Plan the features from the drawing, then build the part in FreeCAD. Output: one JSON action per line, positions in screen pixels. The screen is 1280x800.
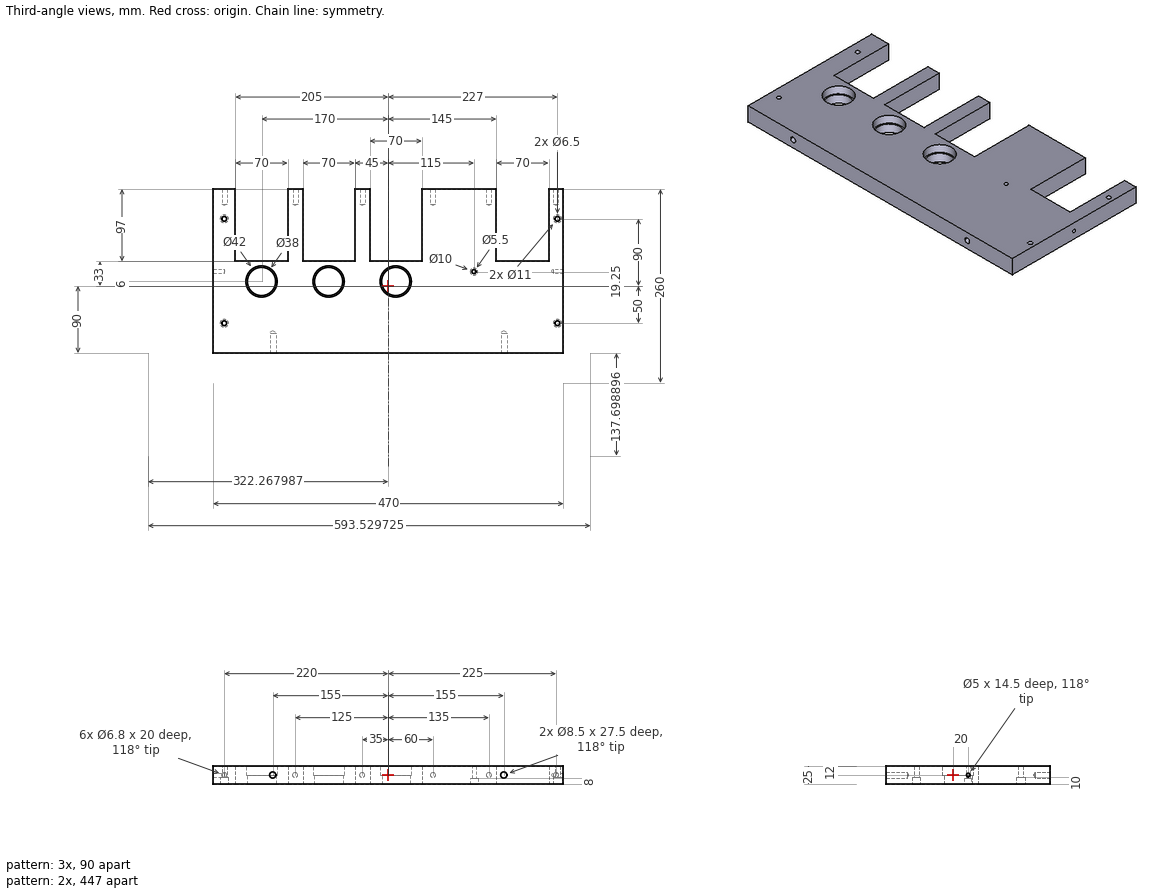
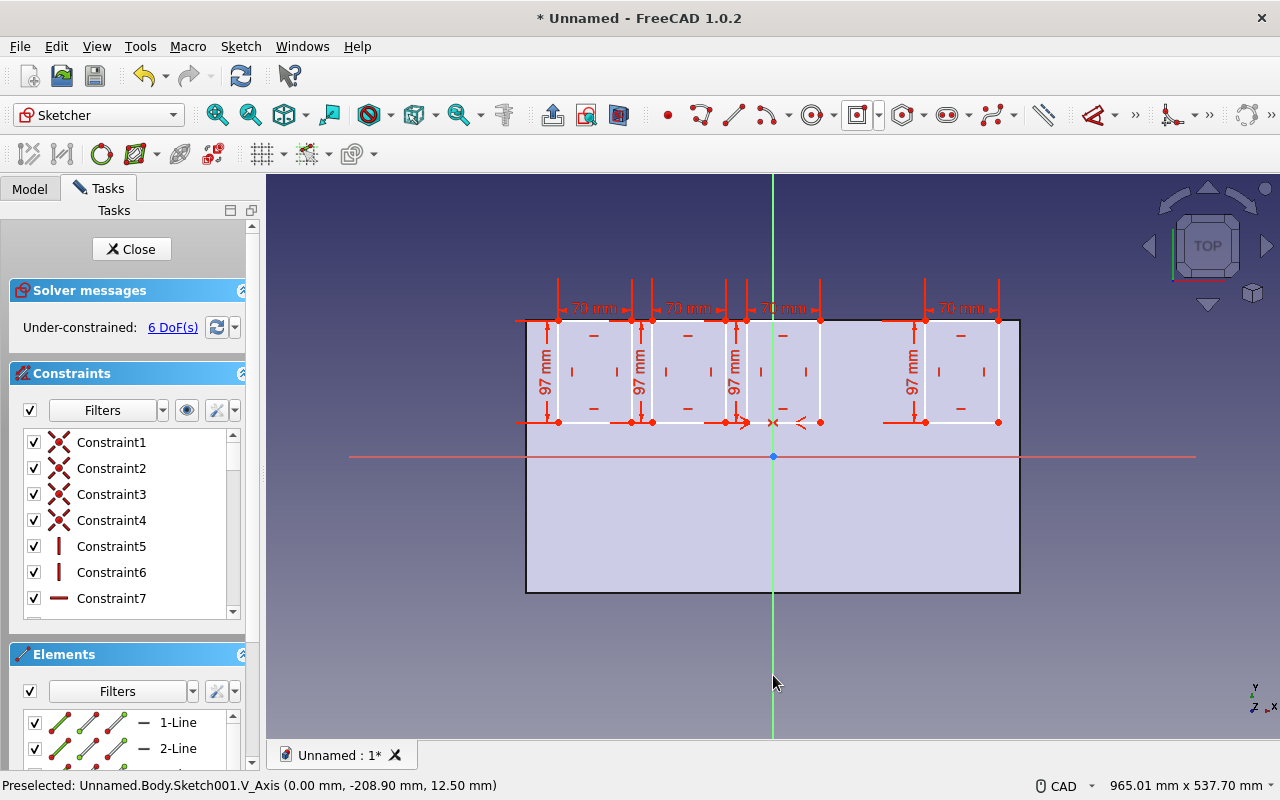
{"action": "left_click", "coordinate": [1092, 116]}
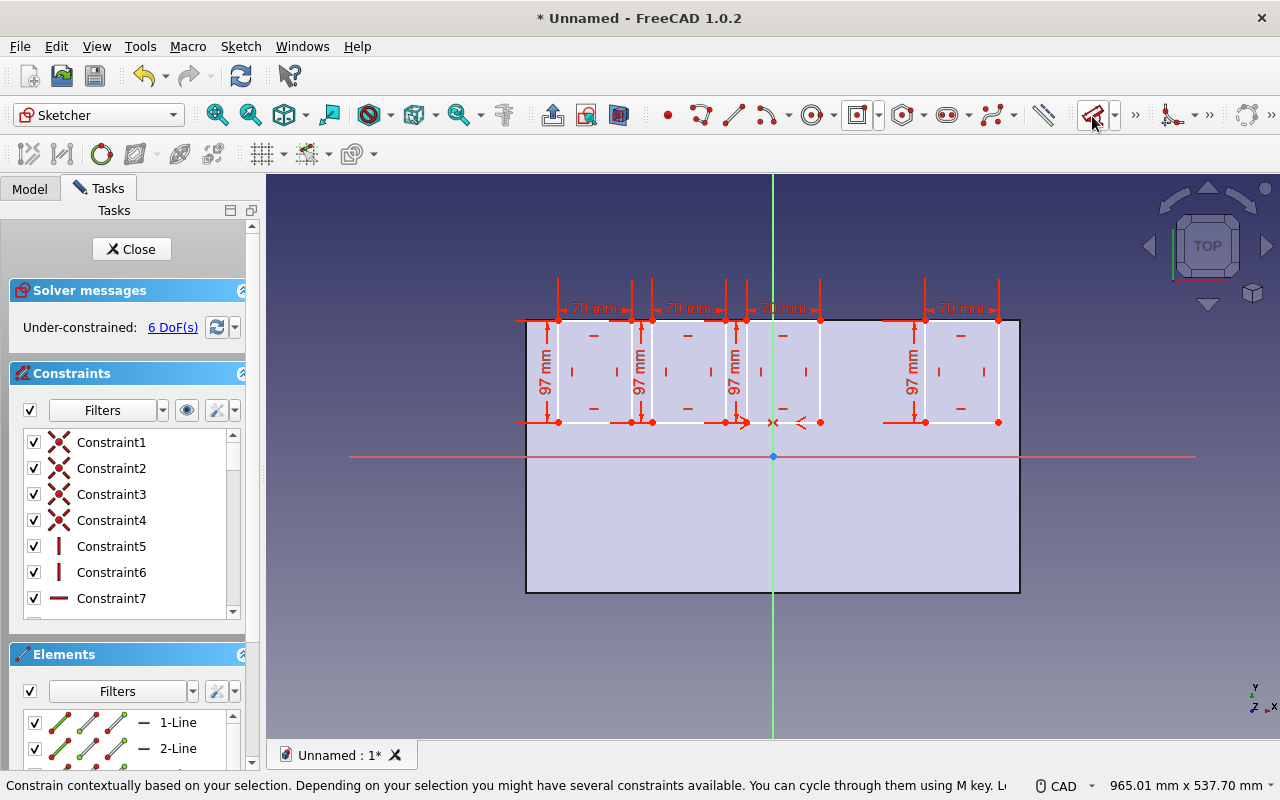
{"action": "left_click", "coordinate": [558, 423]}
{"action": "left_click", "coordinate": [524, 440]}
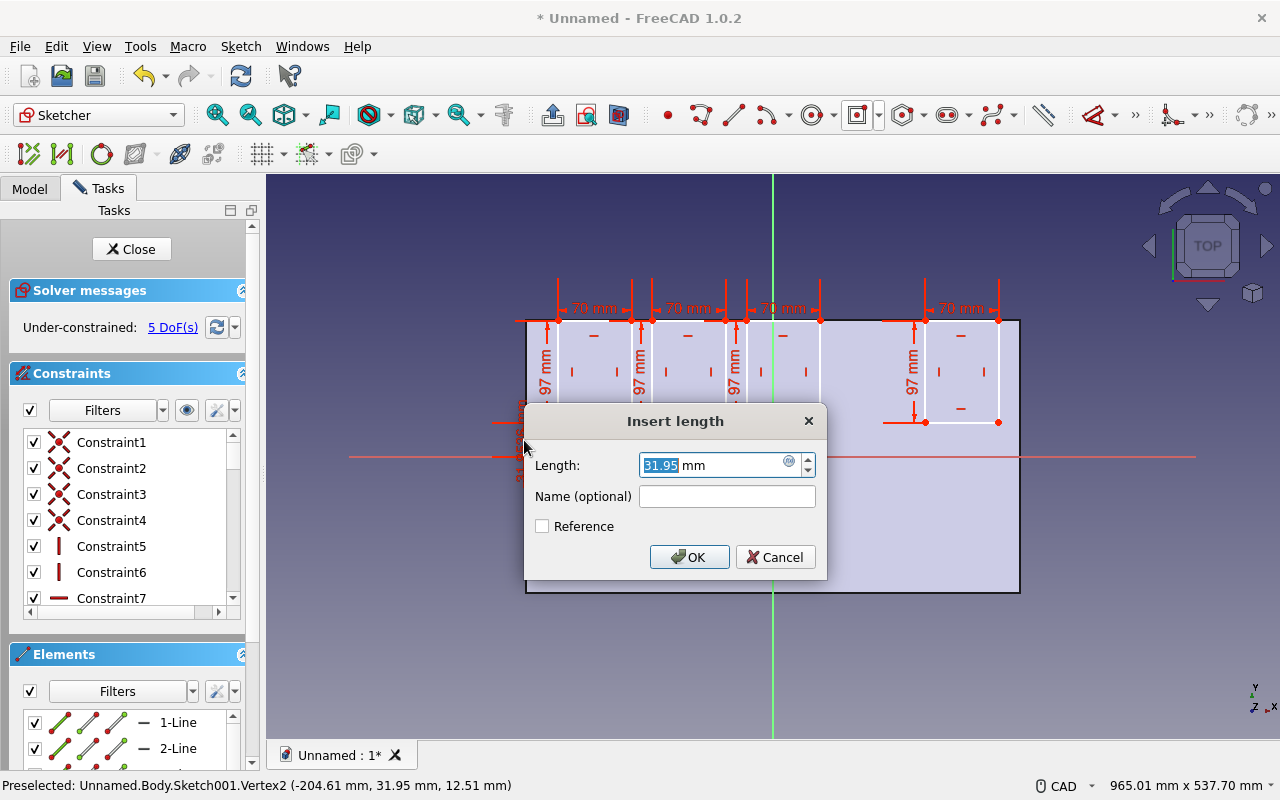
{"action": "type", "text": "33"}
{"action": "key", "text": "Return"}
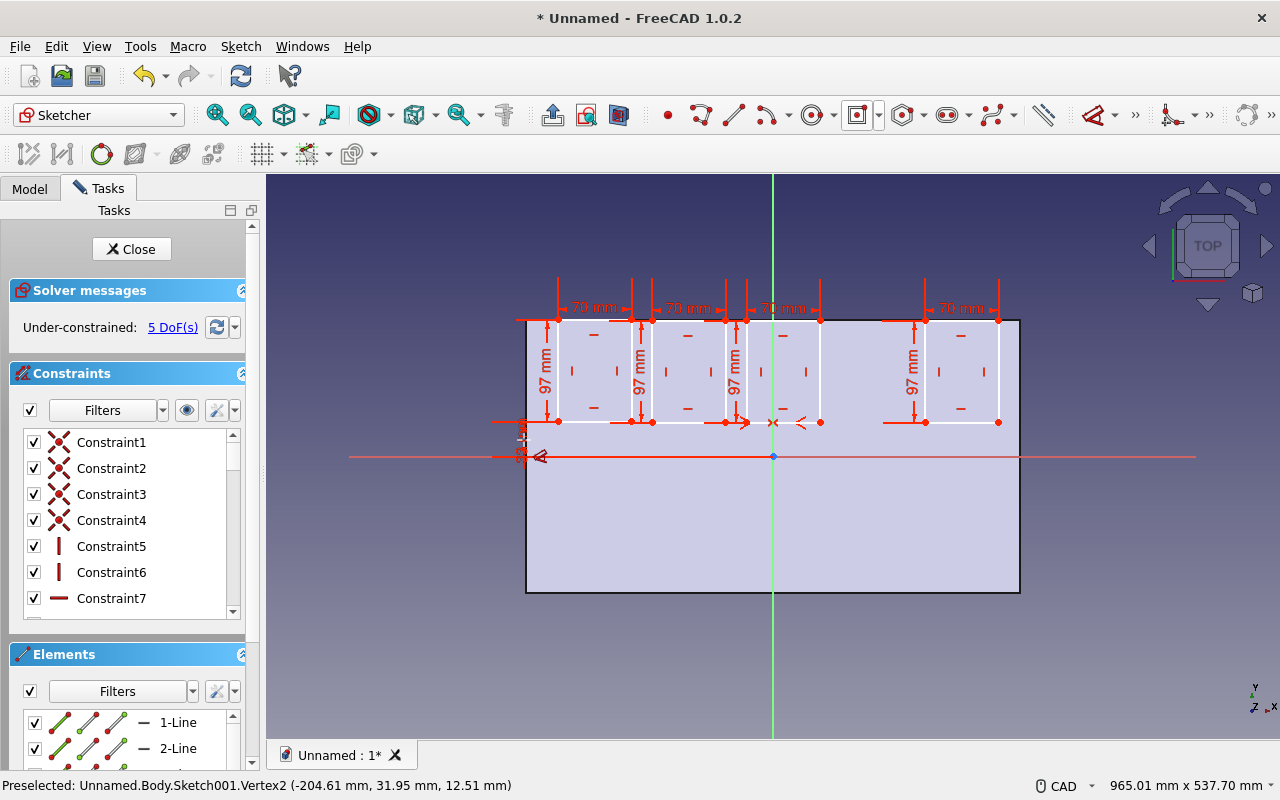
{"action": "left_click", "coordinate": [652, 423]}
{"action": "left_click", "coordinate": [618, 440]}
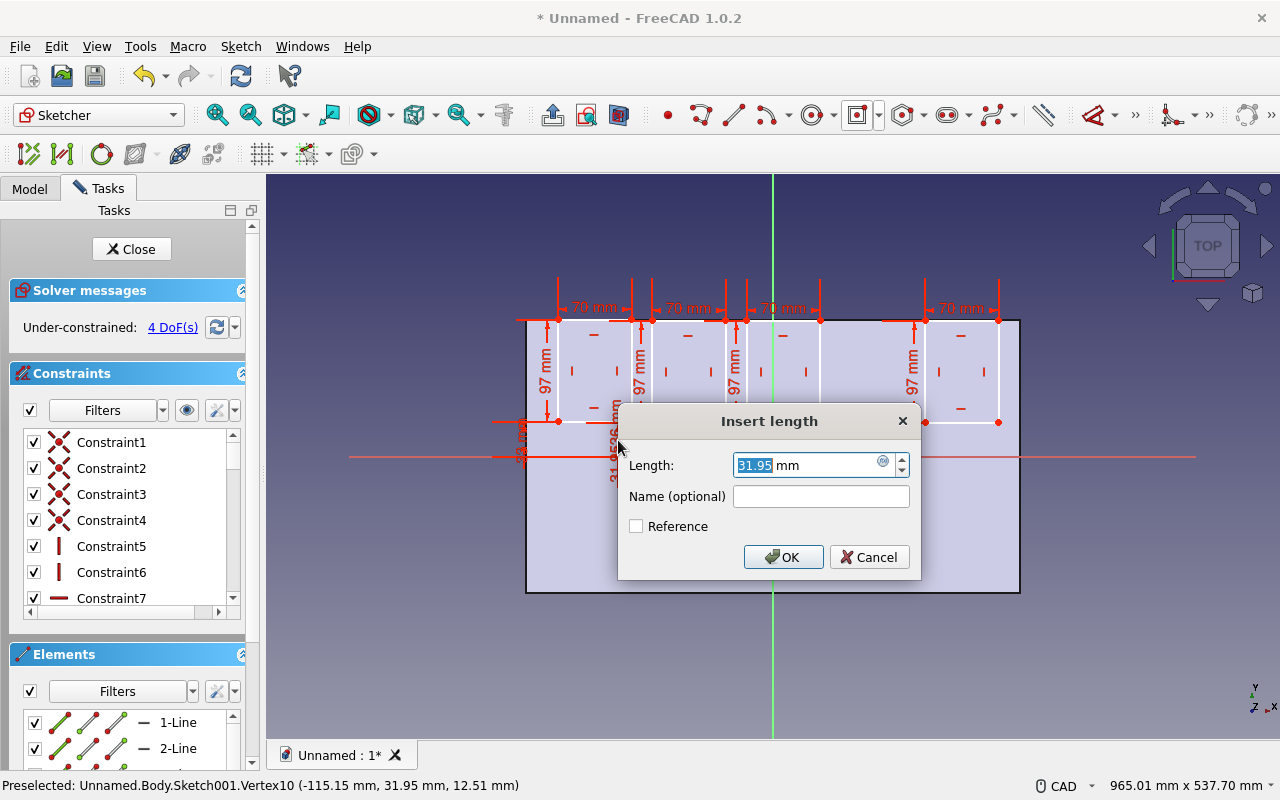
{"action": "type", "text": "33"}
{"action": "key", "text": "Return"}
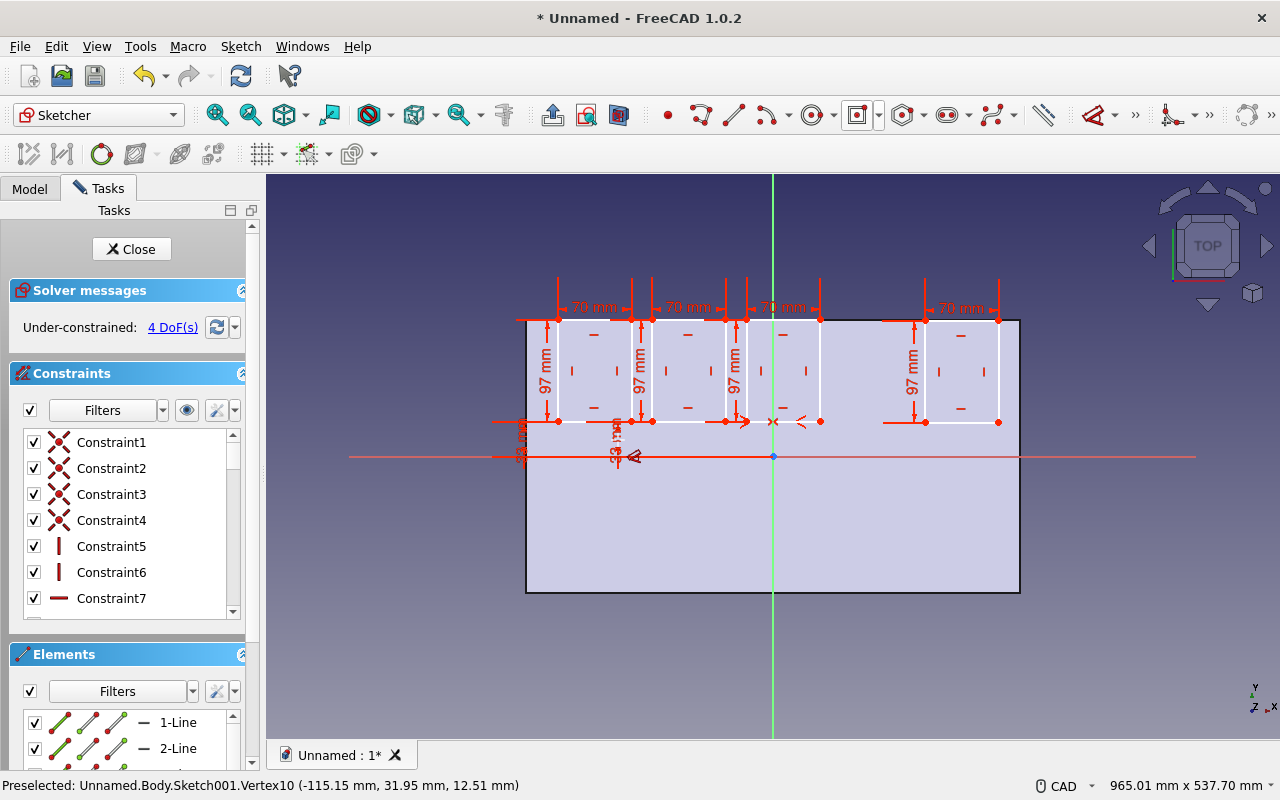
{"action": "left_click", "coordinate": [726, 422]}
{"action": "left_click", "coordinate": [749, 490]}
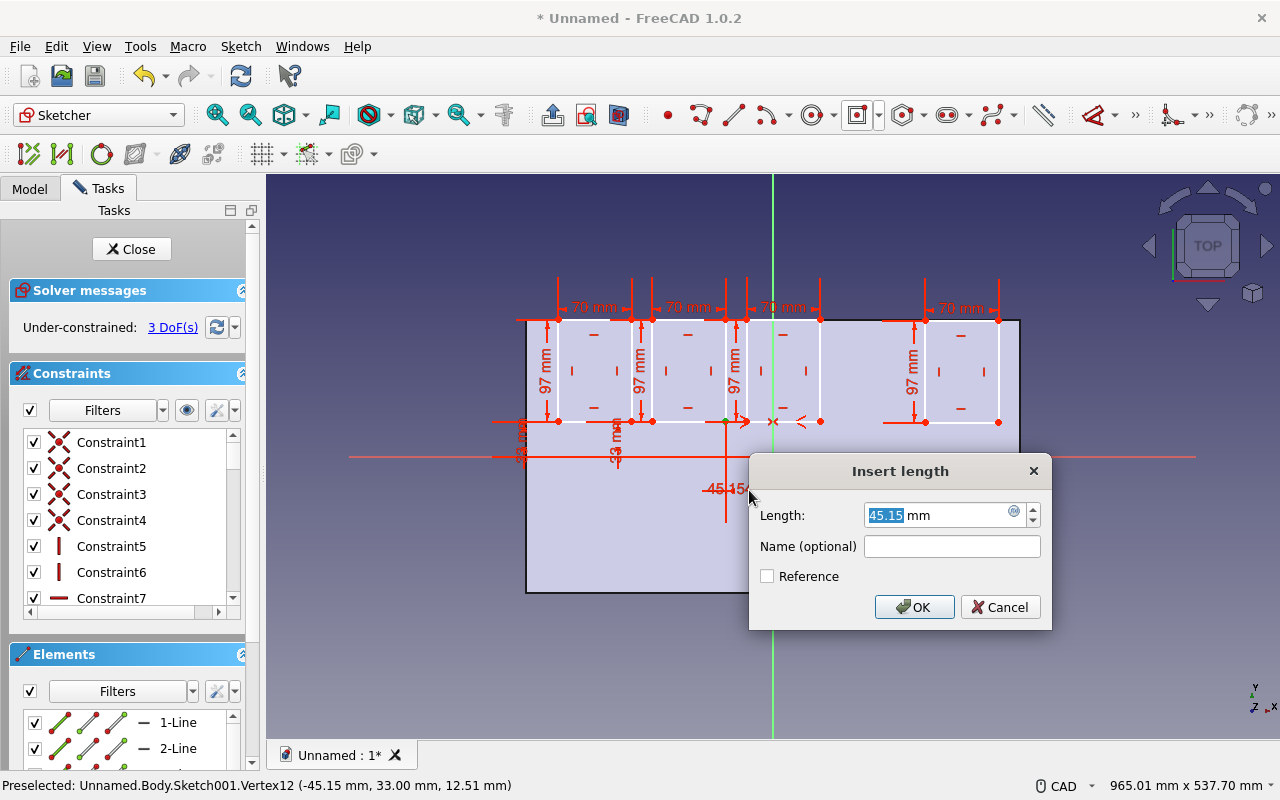
{"action": "type", "text": "45"}
{"action": "key", "text": "Return"}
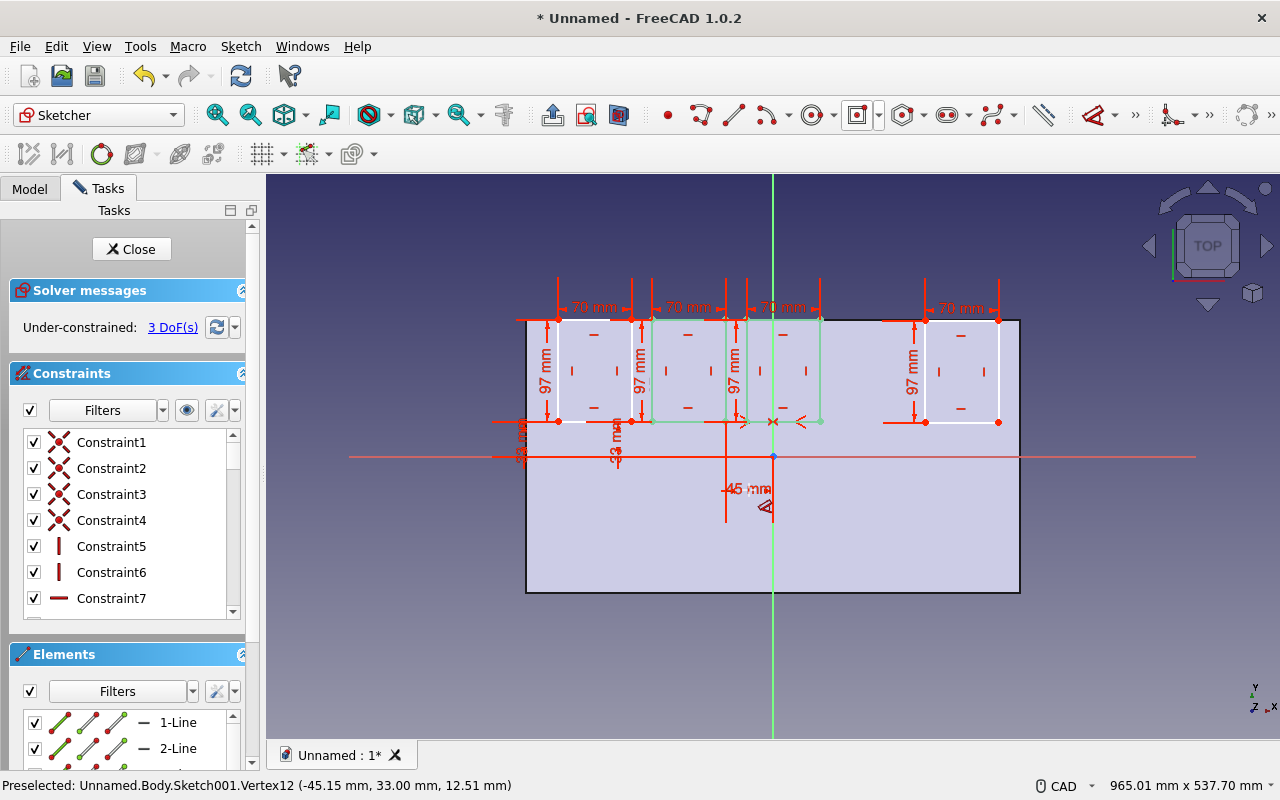
{"action": "left_click", "coordinate": [925, 423]}
{"action": "left_click", "coordinate": [959, 440]}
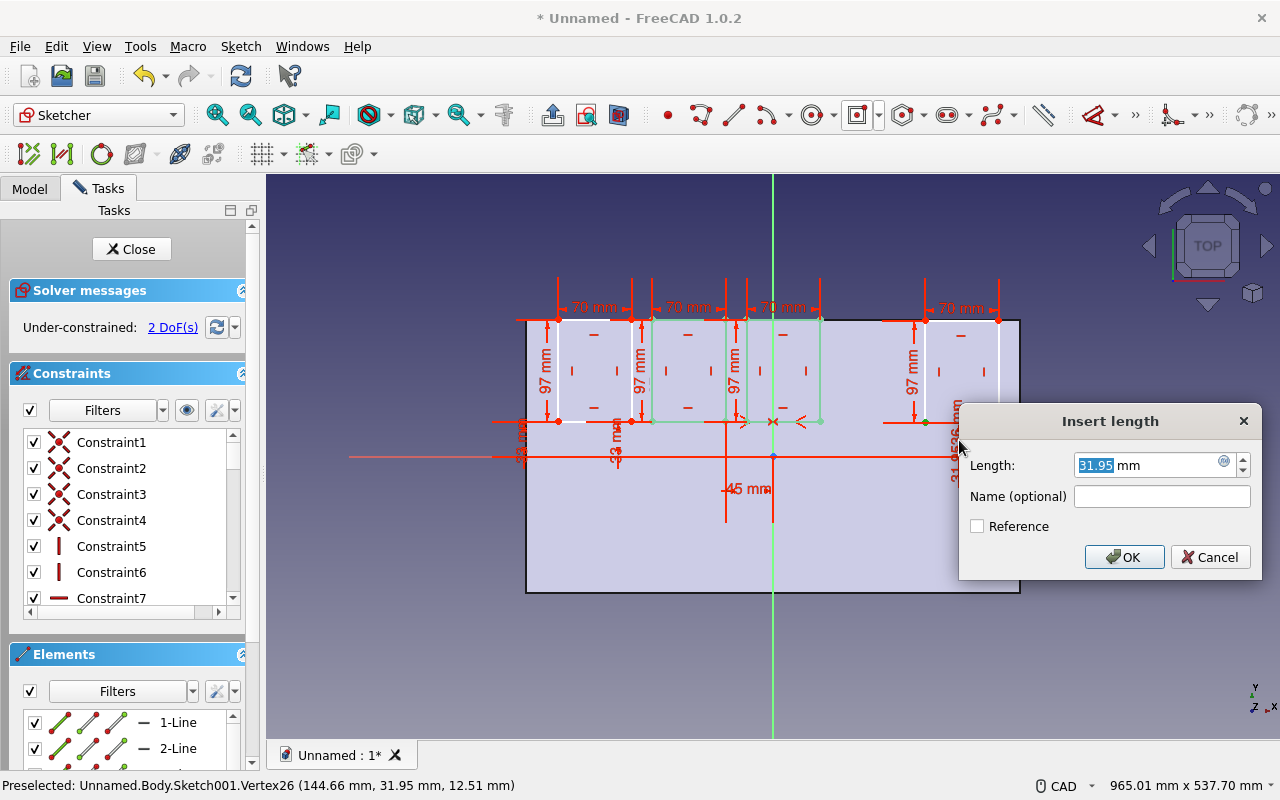
{"action": "type", "text": "33"}
{"action": "key", "text": "Return"}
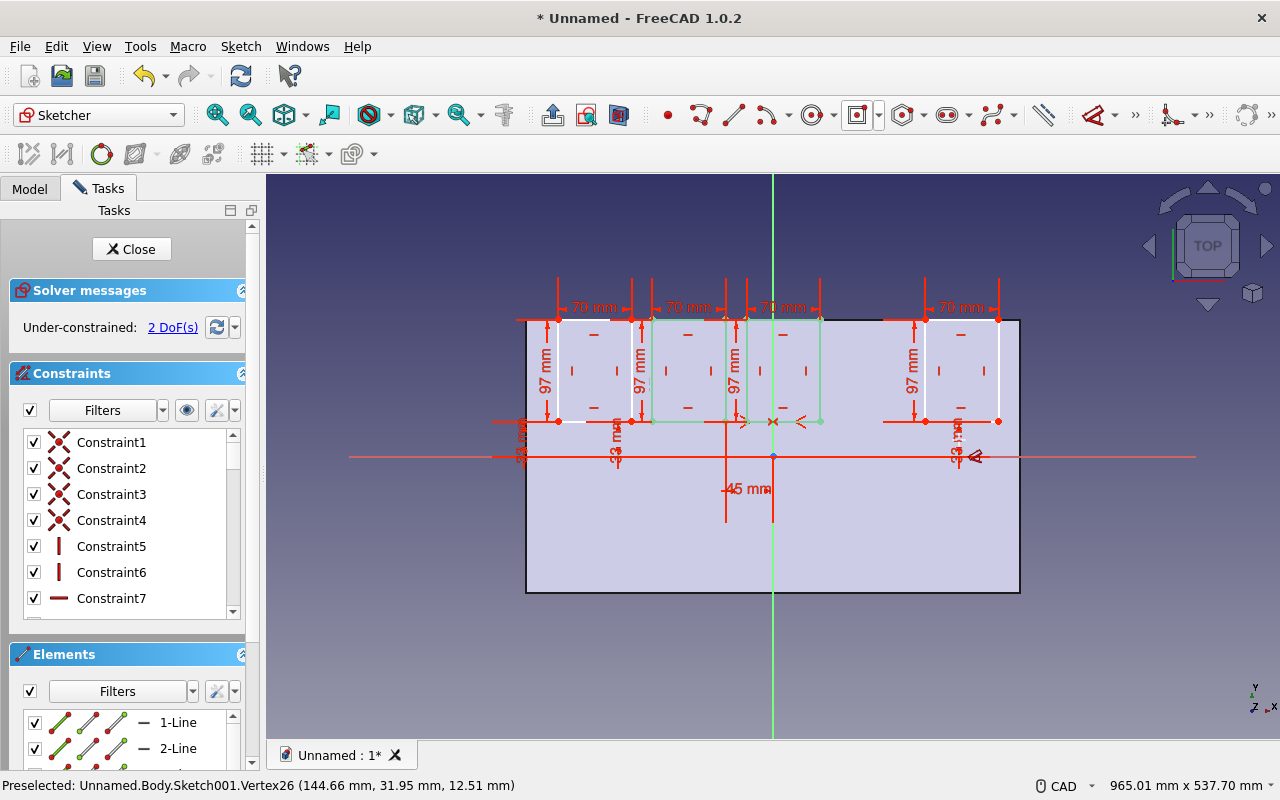
{"action": "left_click", "coordinate": [558, 320]}
{"action": "left_click", "coordinate": [666, 490]}